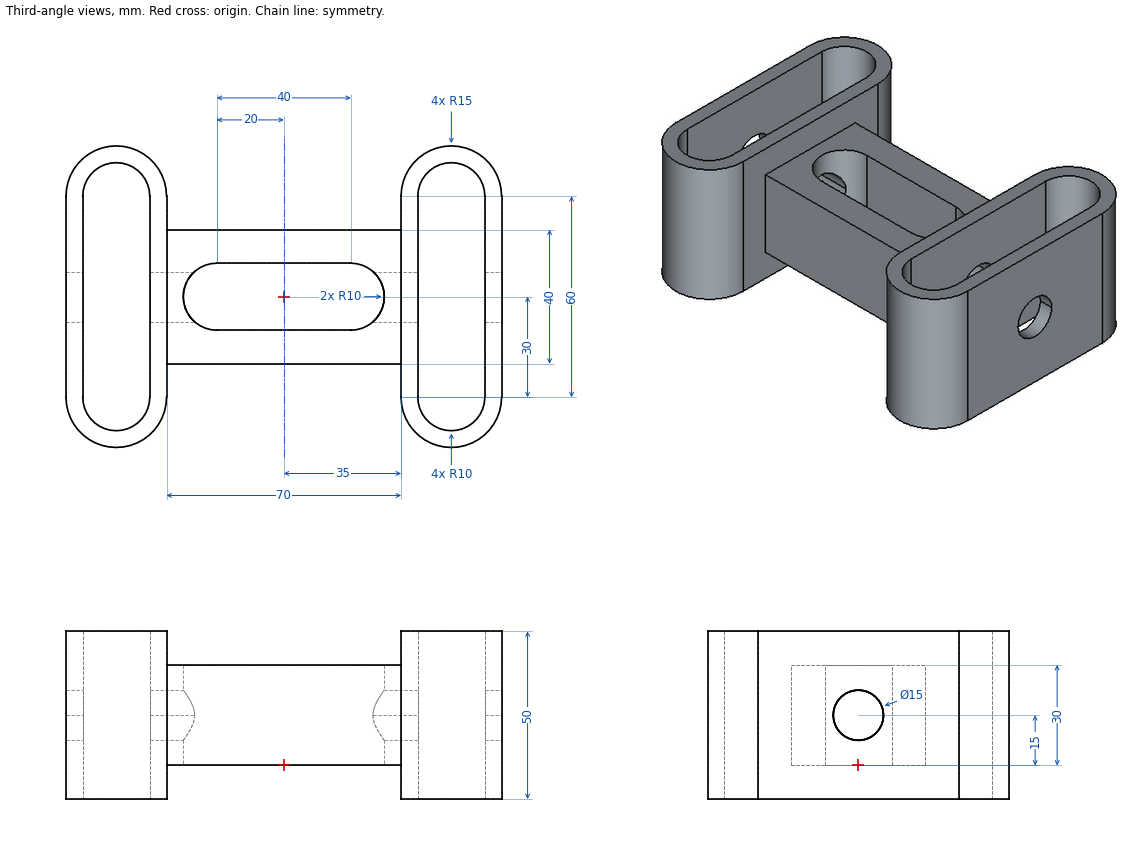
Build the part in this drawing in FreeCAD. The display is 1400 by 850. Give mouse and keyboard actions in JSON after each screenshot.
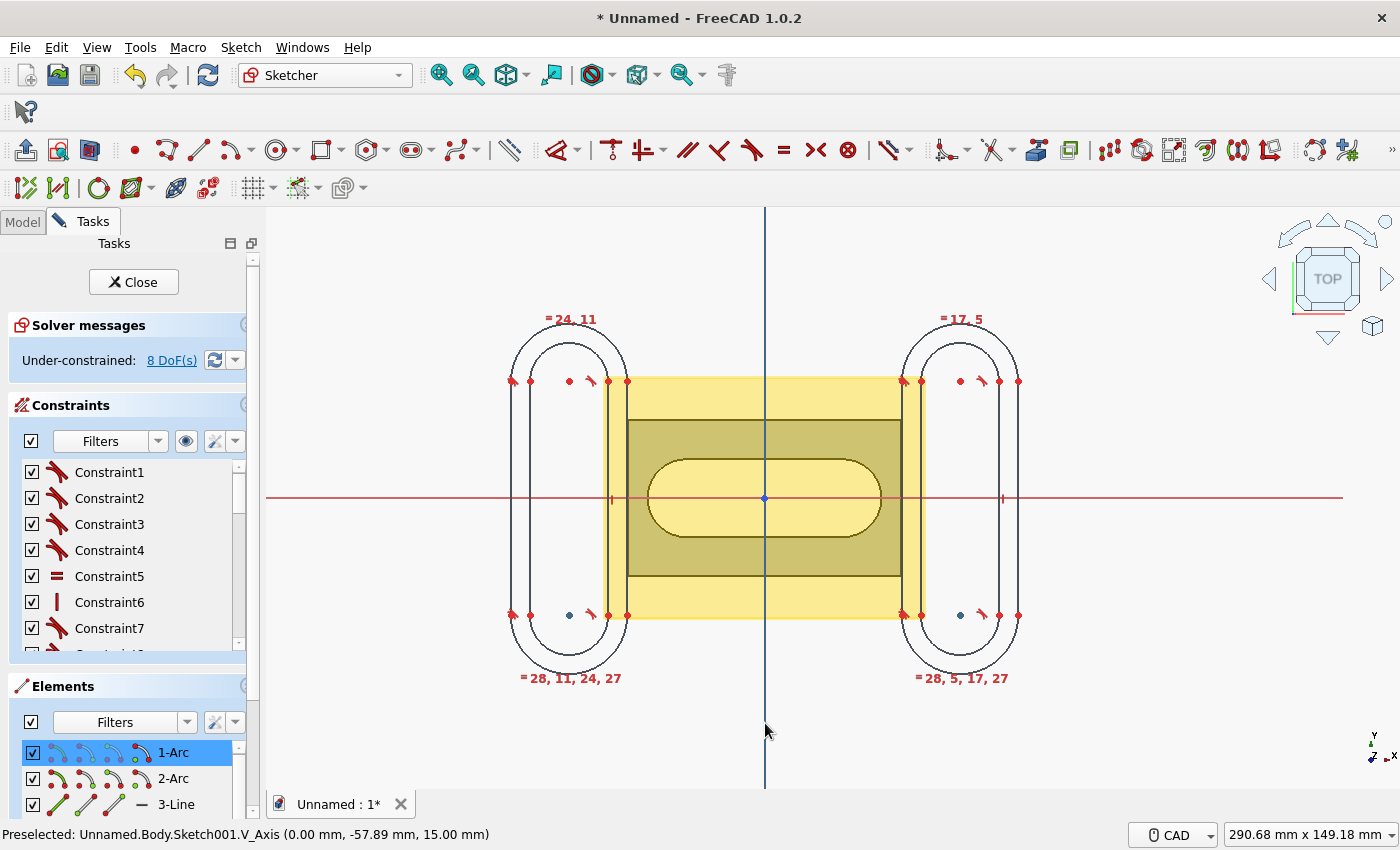
{"action": "key", "text": "s"}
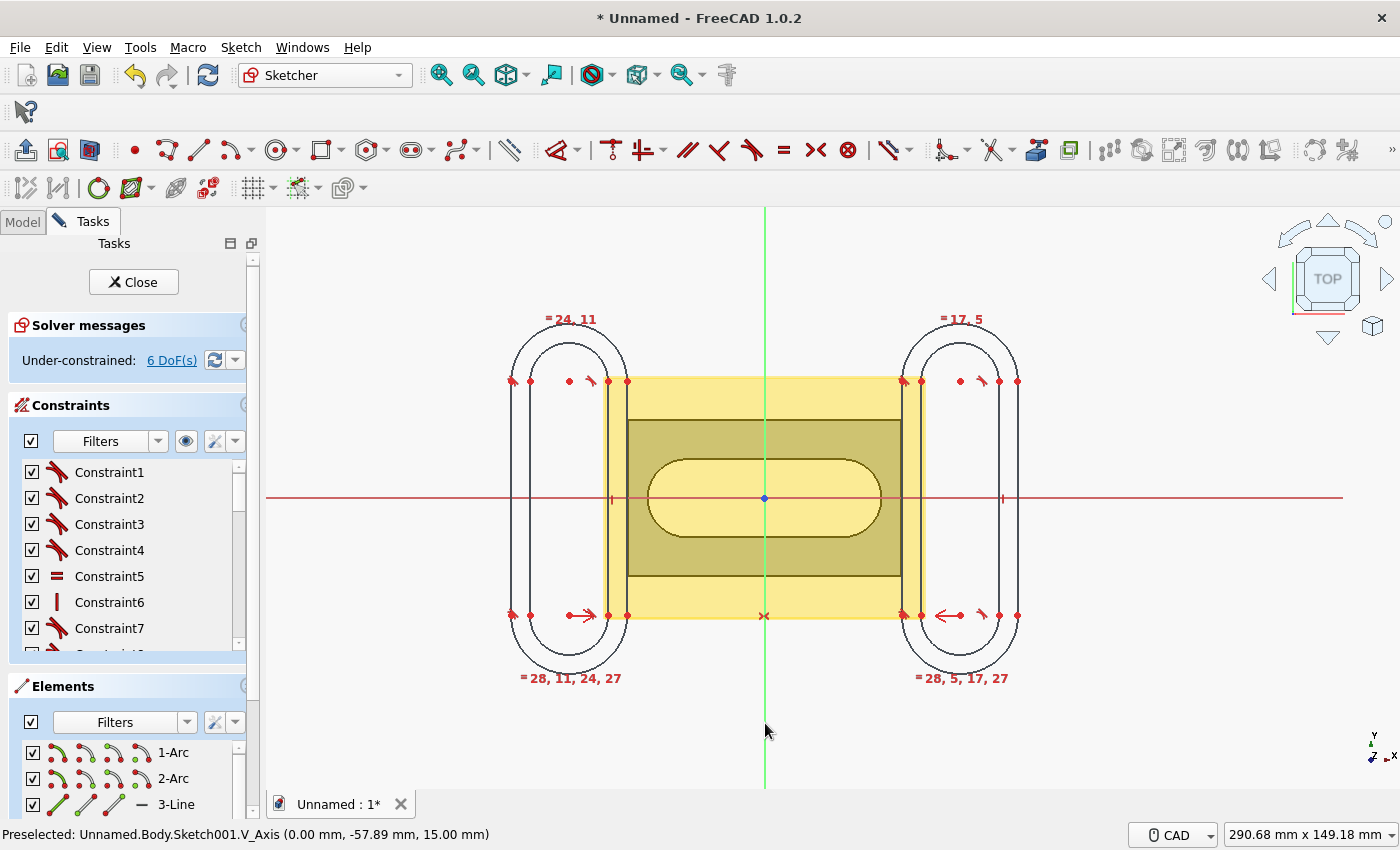
{"action": "key", "text": "d"}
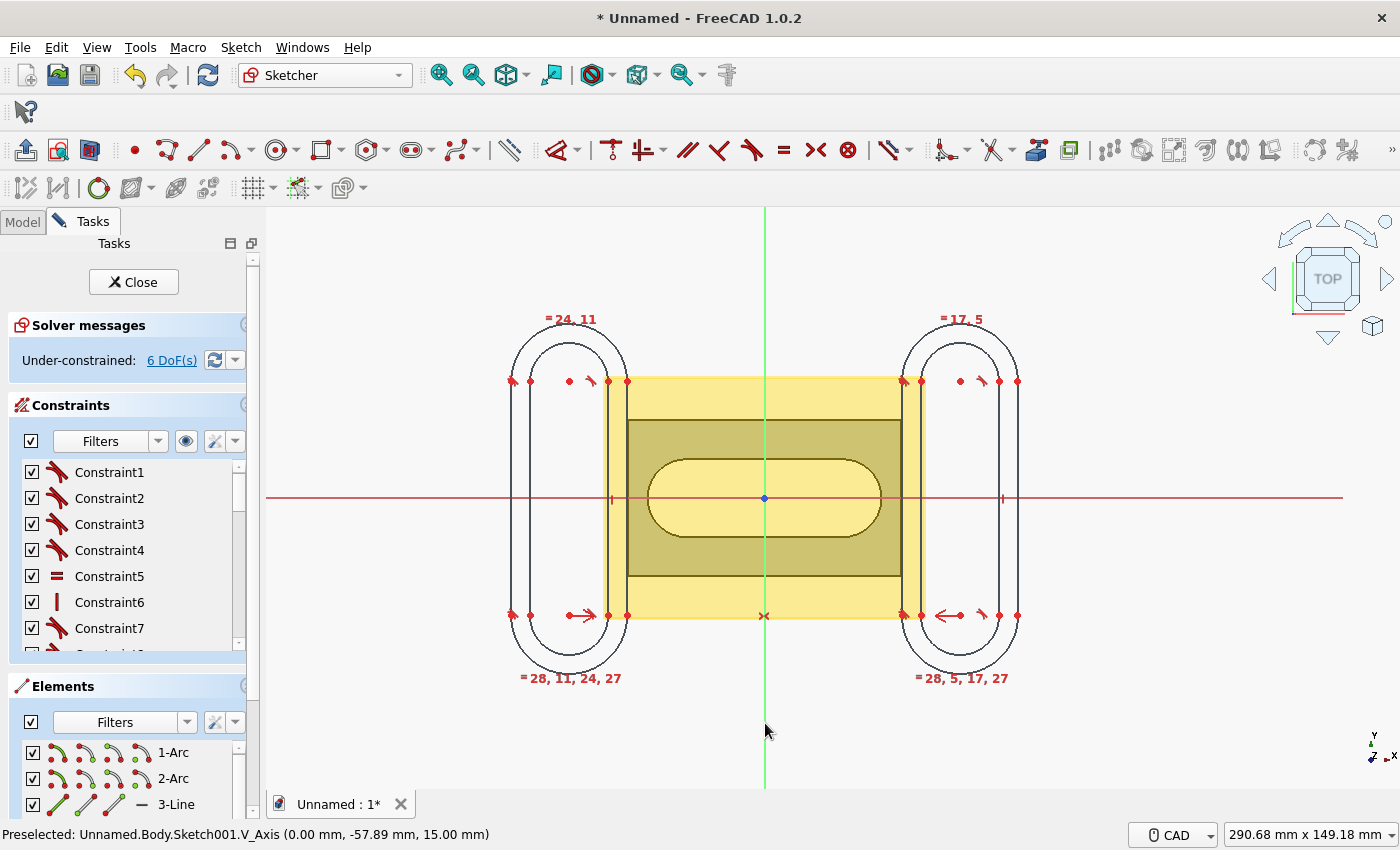
{"action": "left_click", "coordinate": [926, 663]}
{"action": "left_click", "coordinate": [907, 689]}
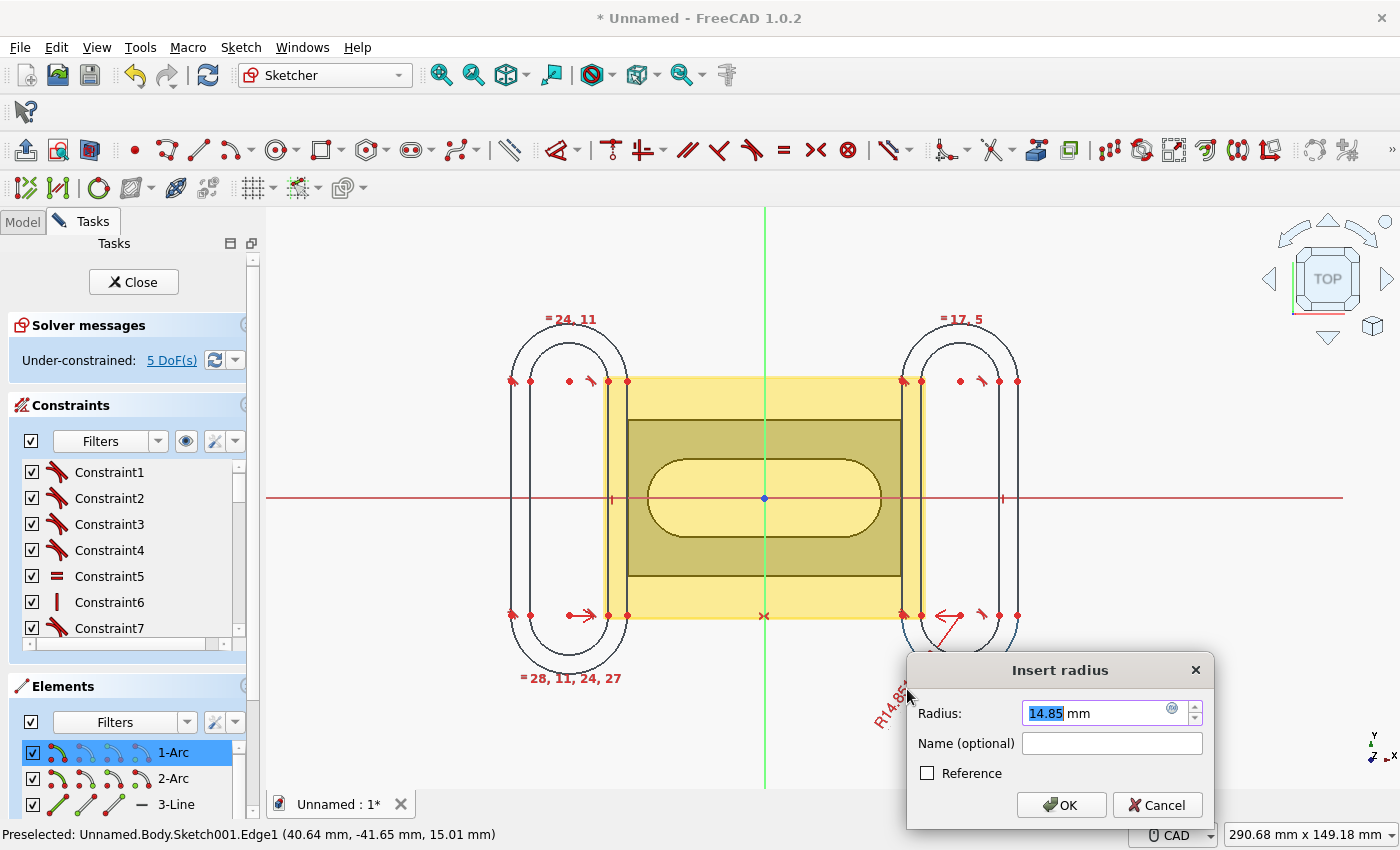
{"action": "type", "text": "15"}
{"action": "key", "text": "Return"}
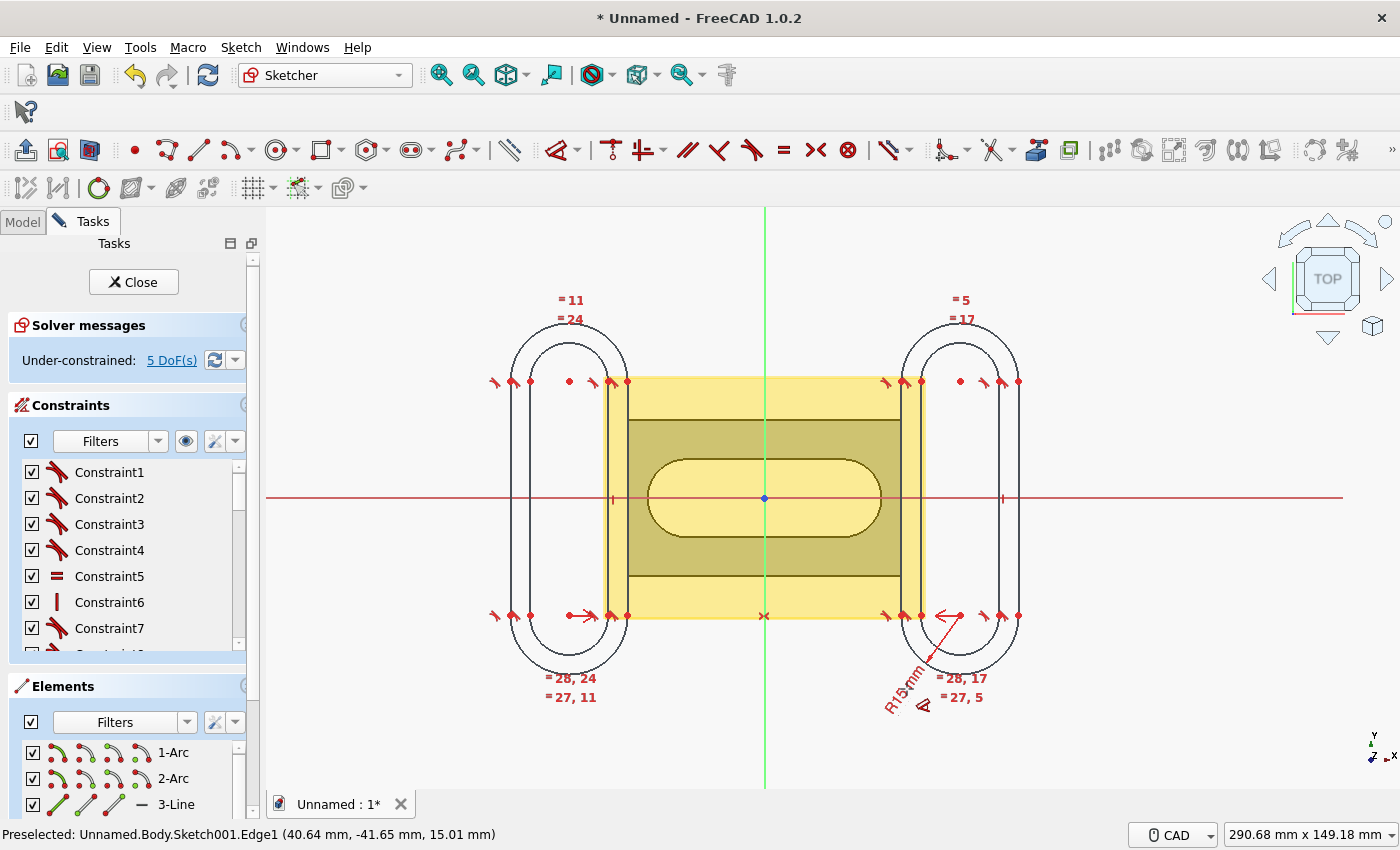
{"action": "left_click", "coordinate": [937, 648]}
{"action": "left_click", "coordinate": [875, 657]}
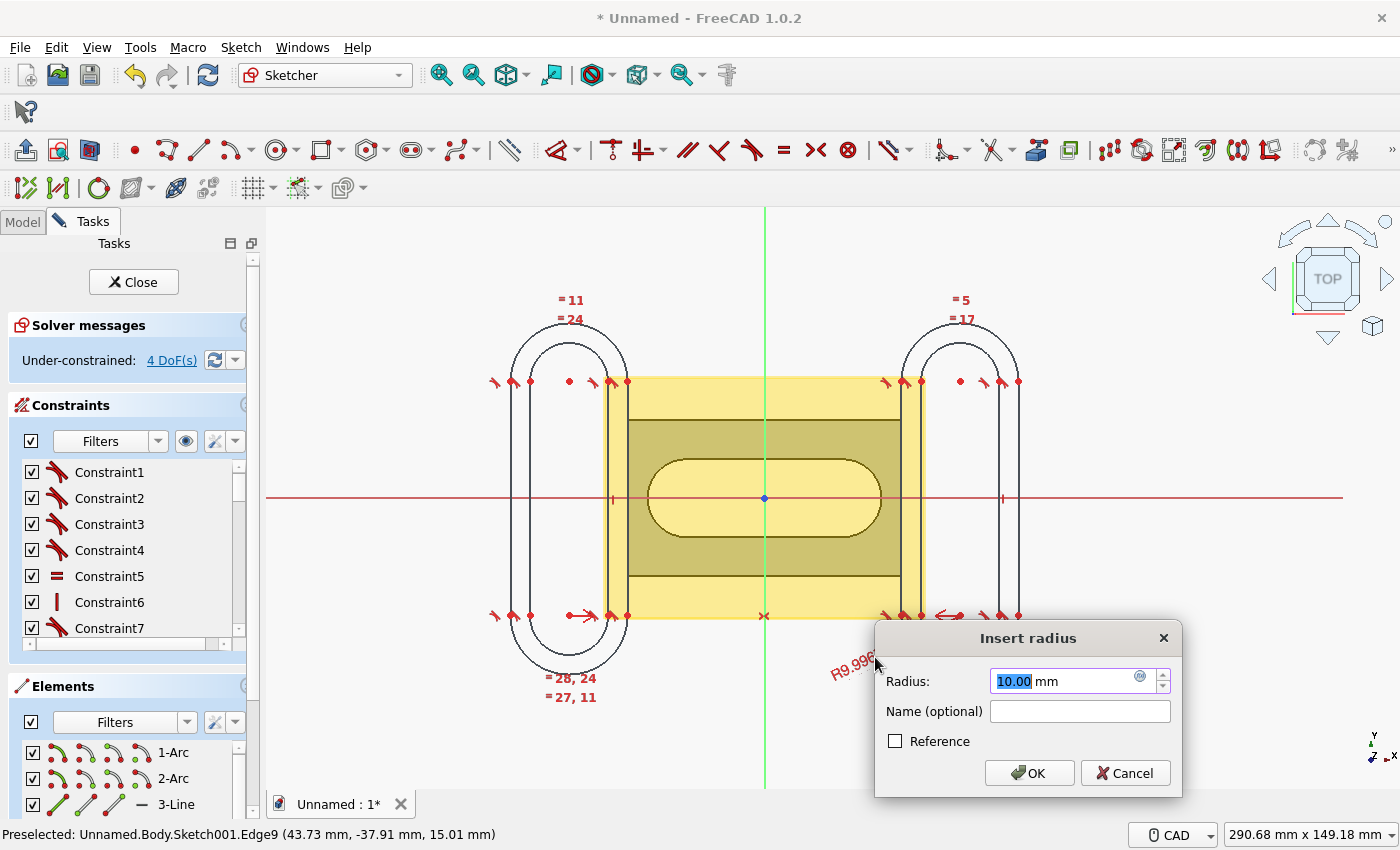
{"action": "type", "text": "10"}
{"action": "key", "text": "Return"}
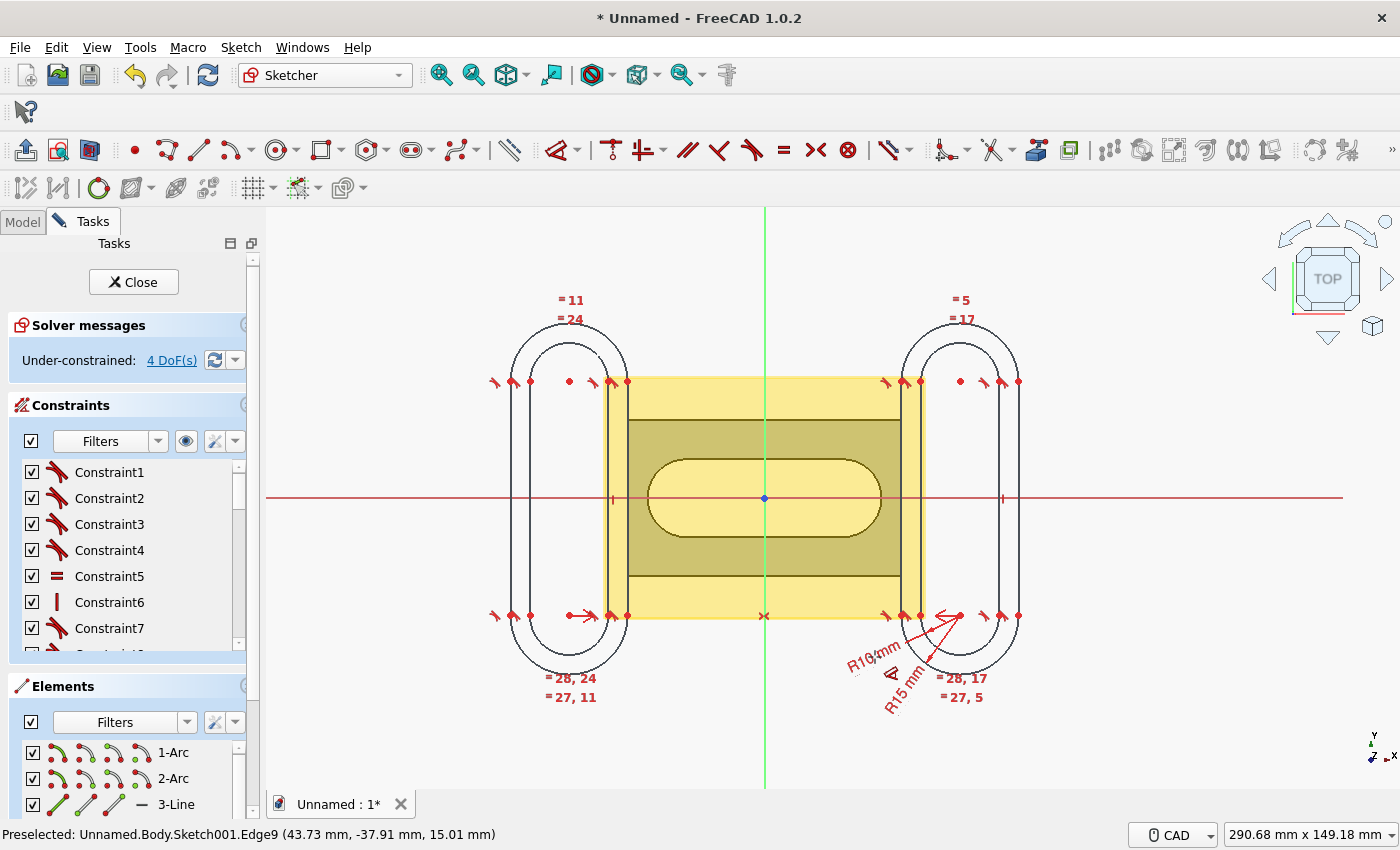
{"action": "left_click", "coordinate": [901, 546]}
{"action": "left_click", "coordinate": [935, 445]}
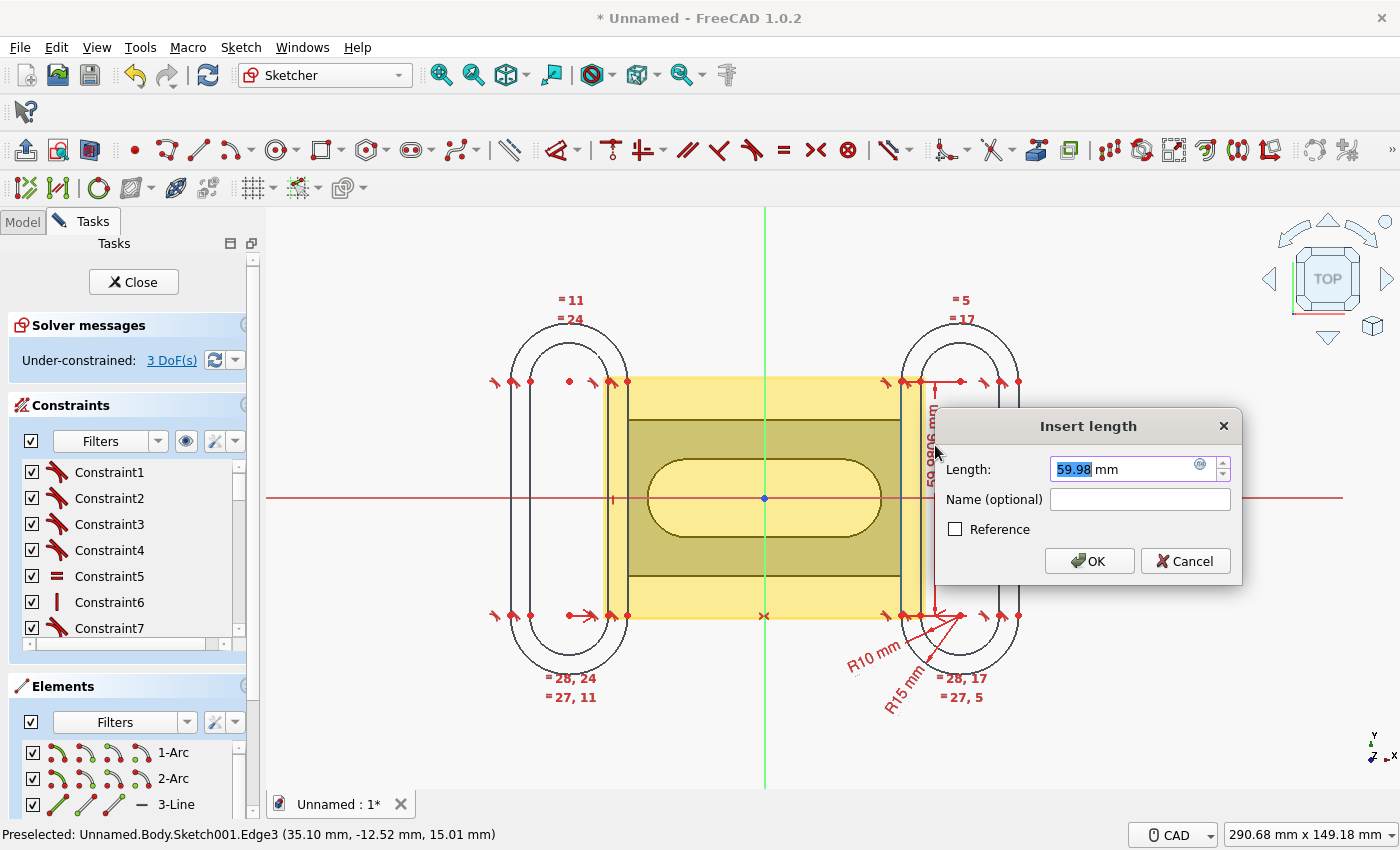
{"action": "type", "text": "60"}
{"action": "key", "text": "Return"}